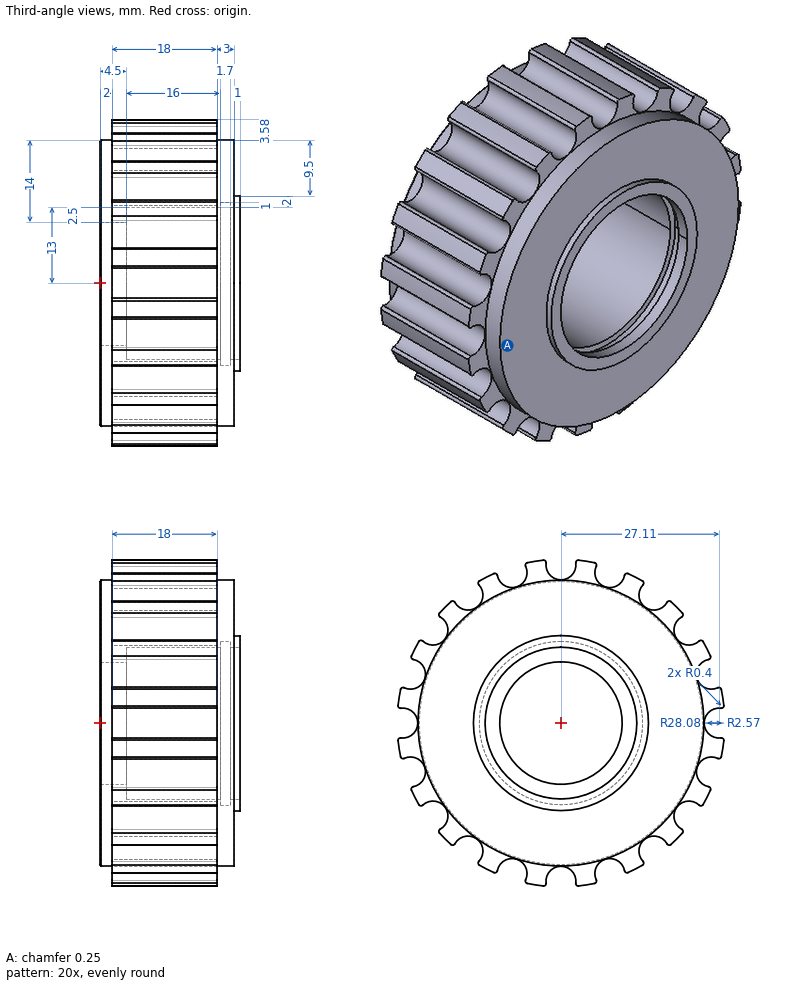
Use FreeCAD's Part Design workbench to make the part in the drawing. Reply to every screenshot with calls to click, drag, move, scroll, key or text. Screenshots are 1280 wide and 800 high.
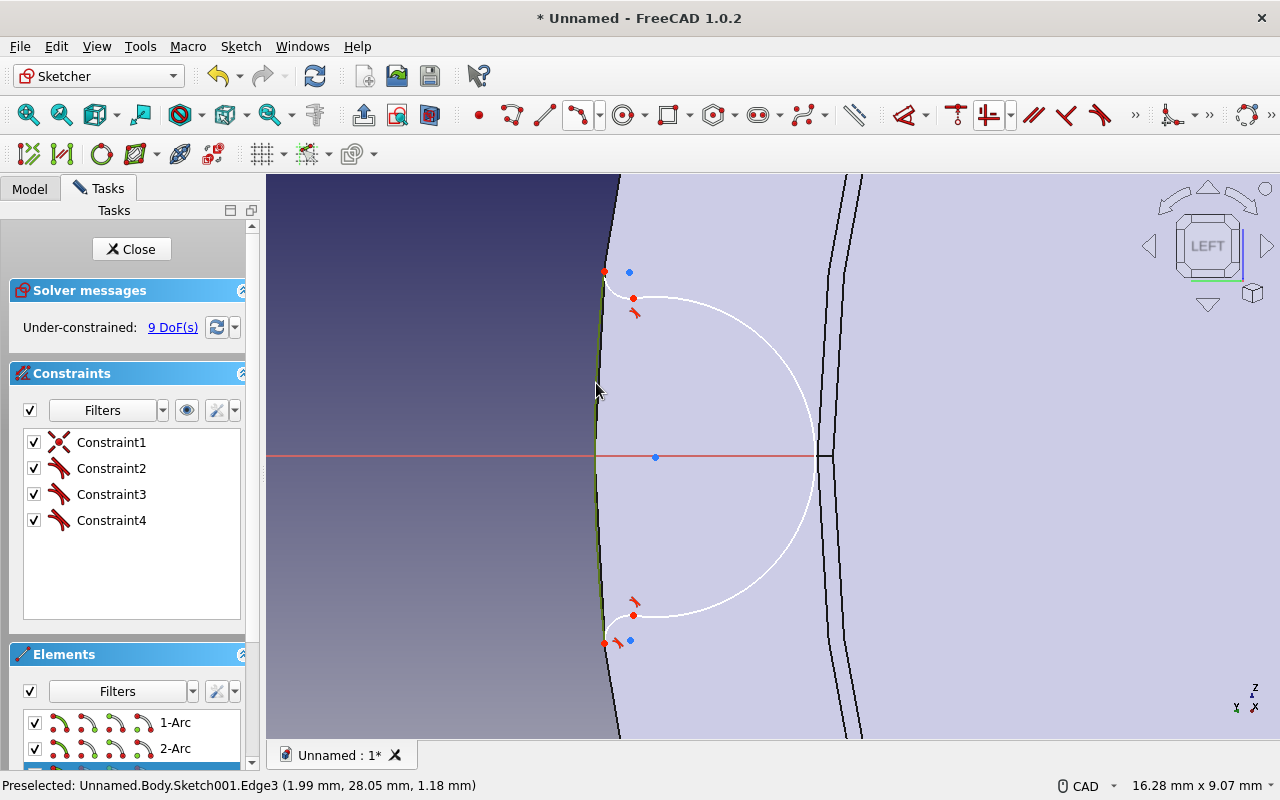
click(620, 297)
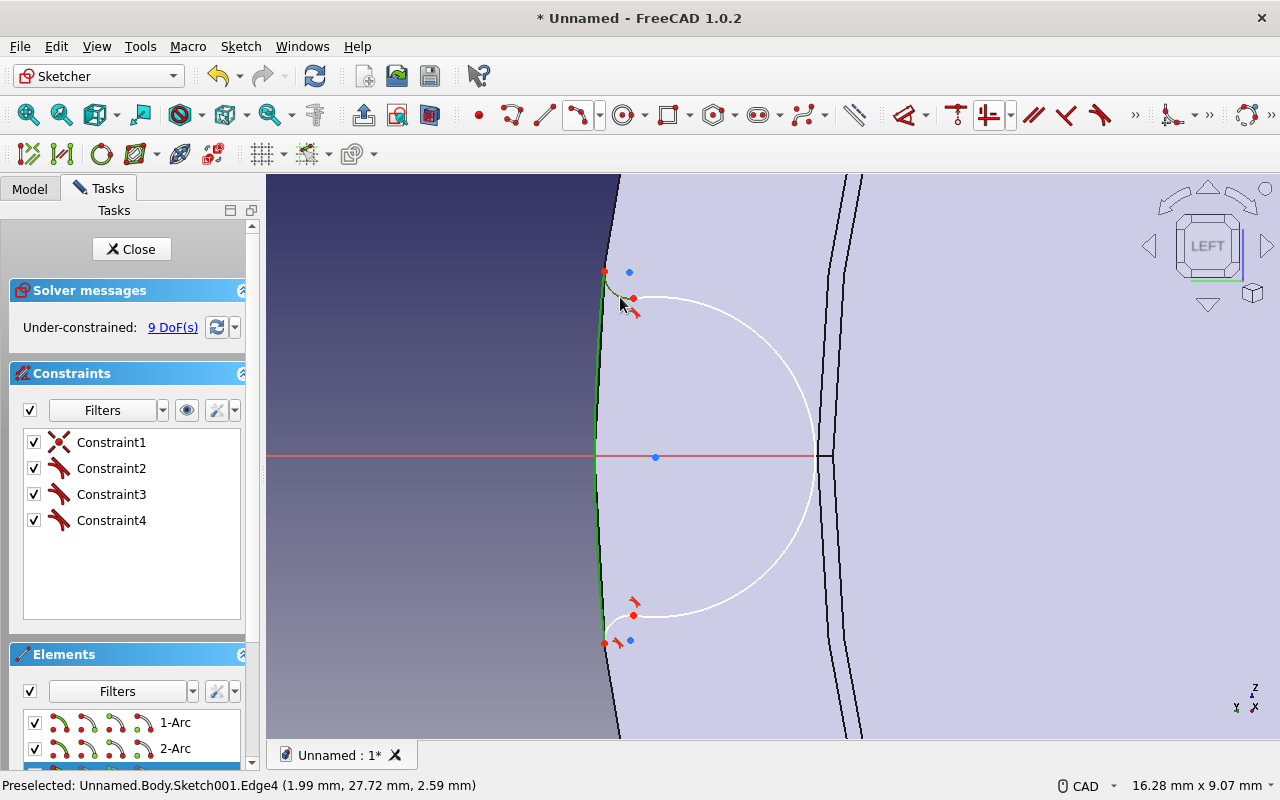
click(1100, 116)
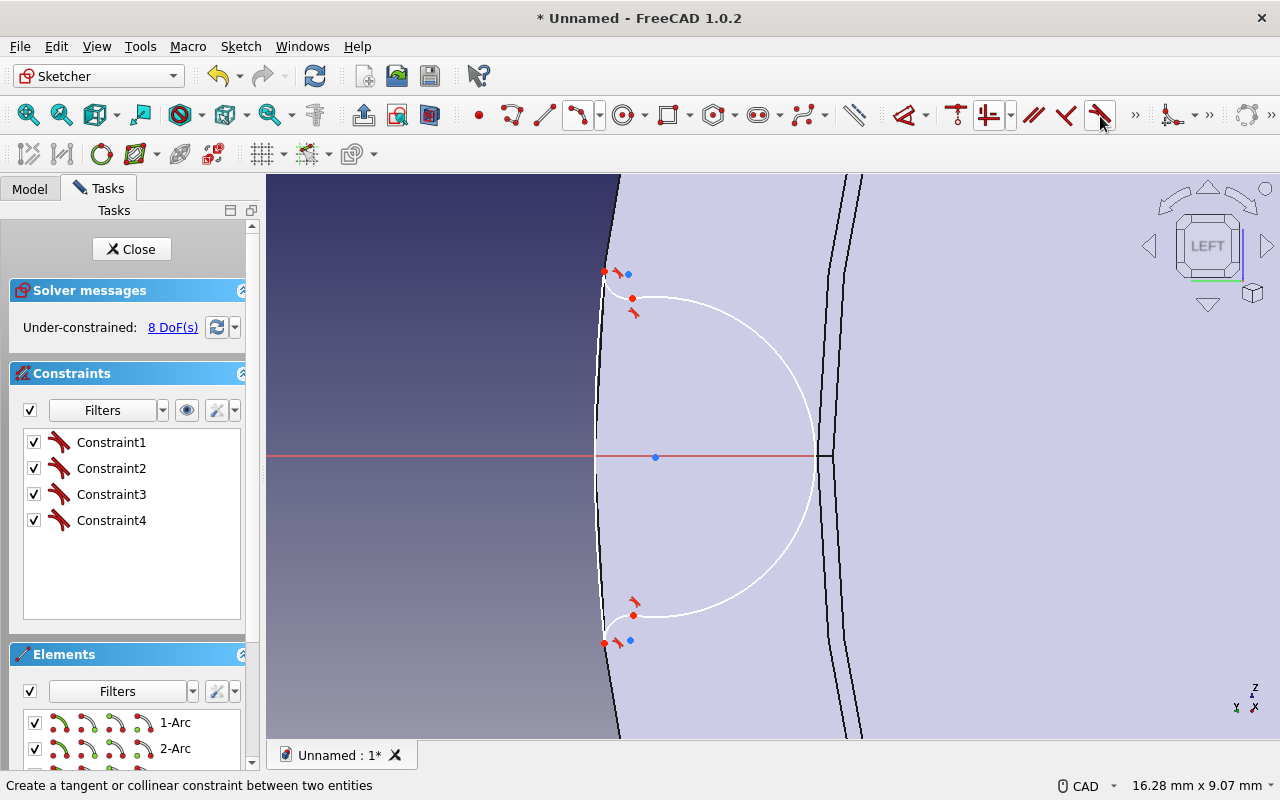
scroll(368, 457, down, 6)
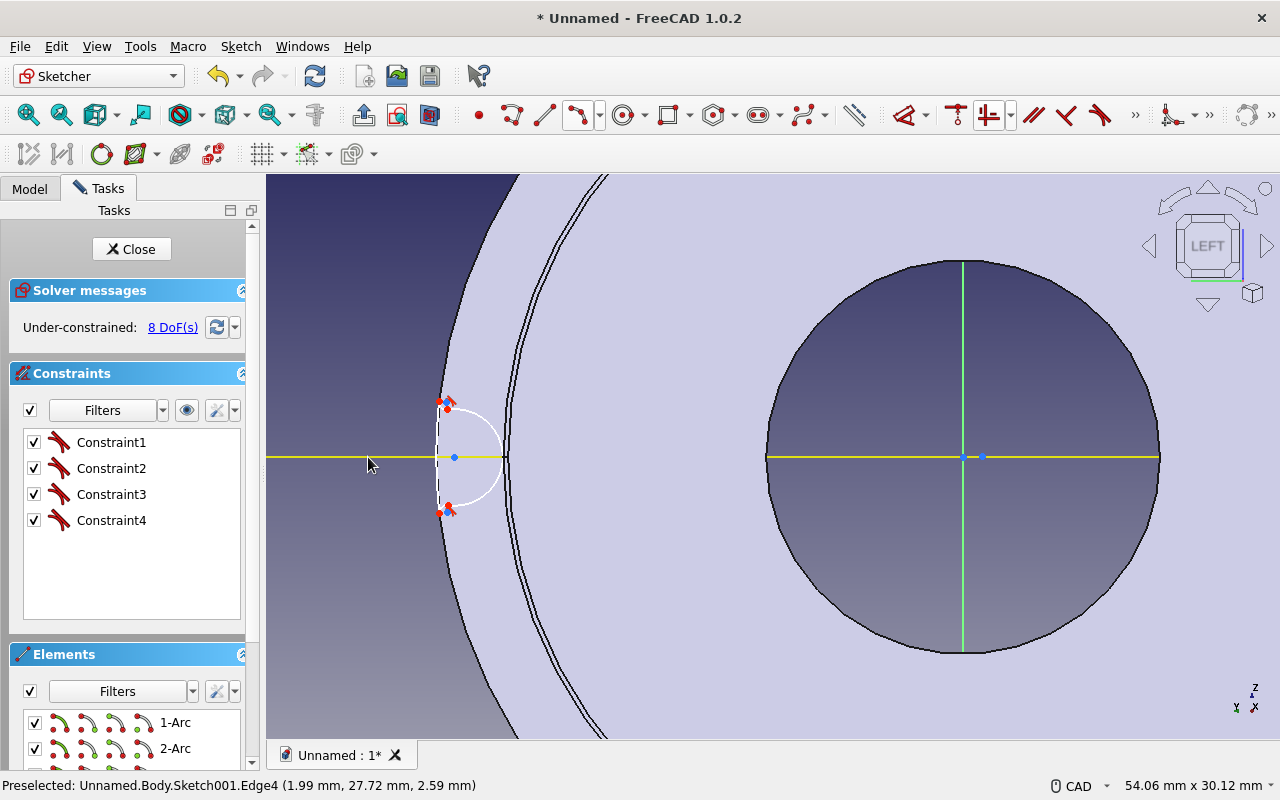
scroll(973, 457, up, 9)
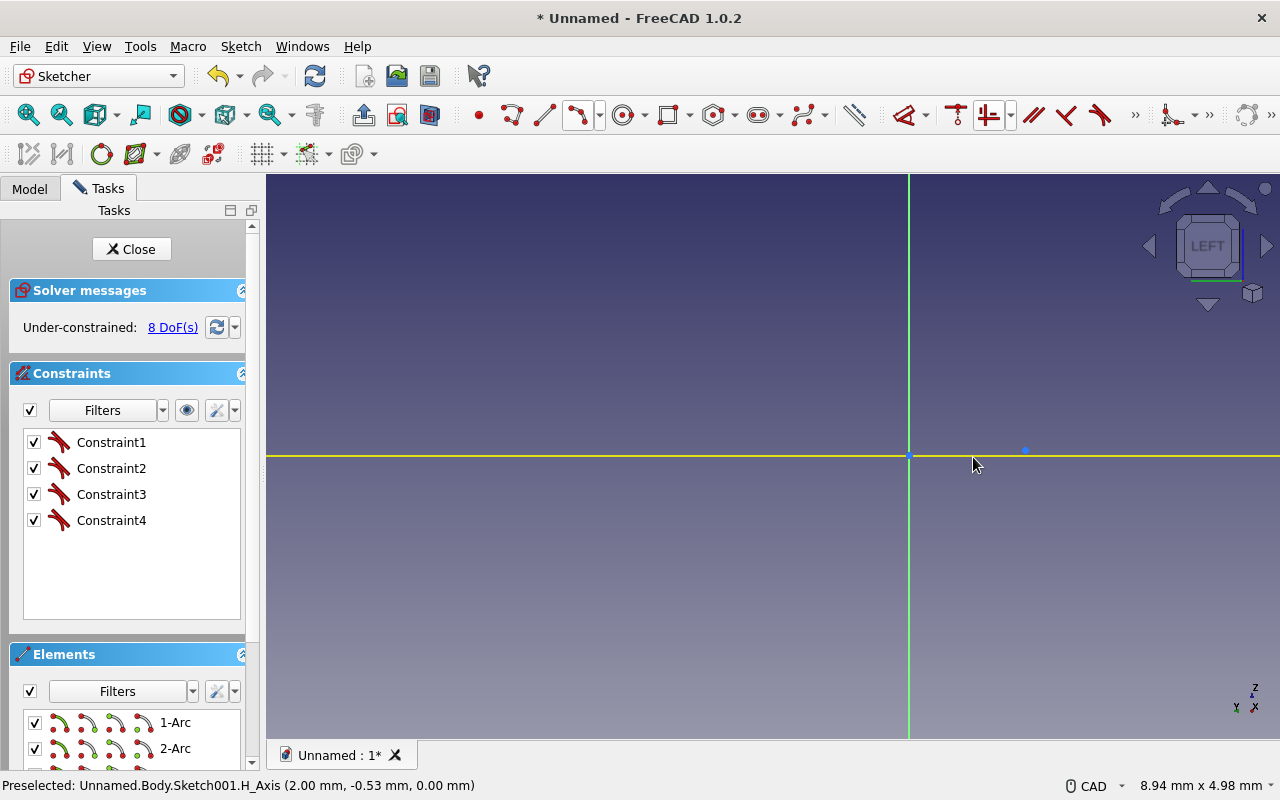
drag(899, 440, 1036, 466)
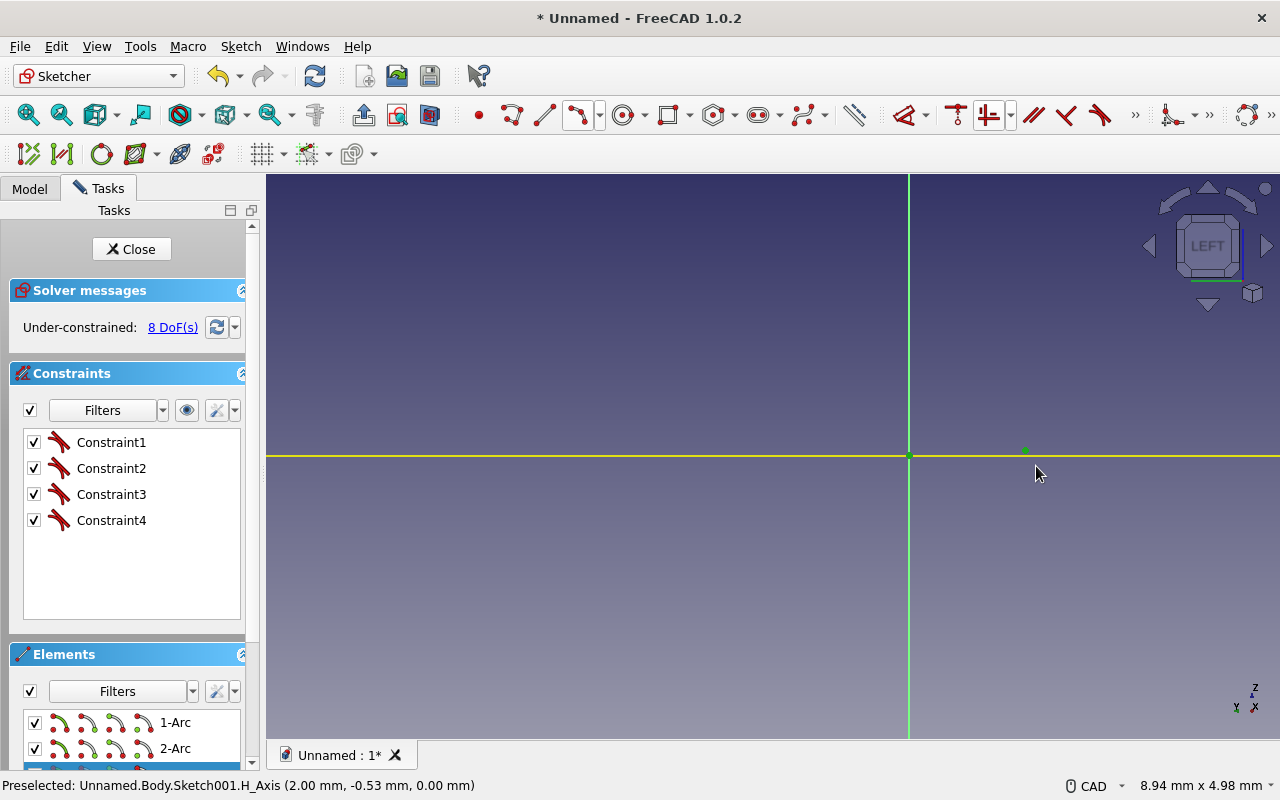
click(956, 116)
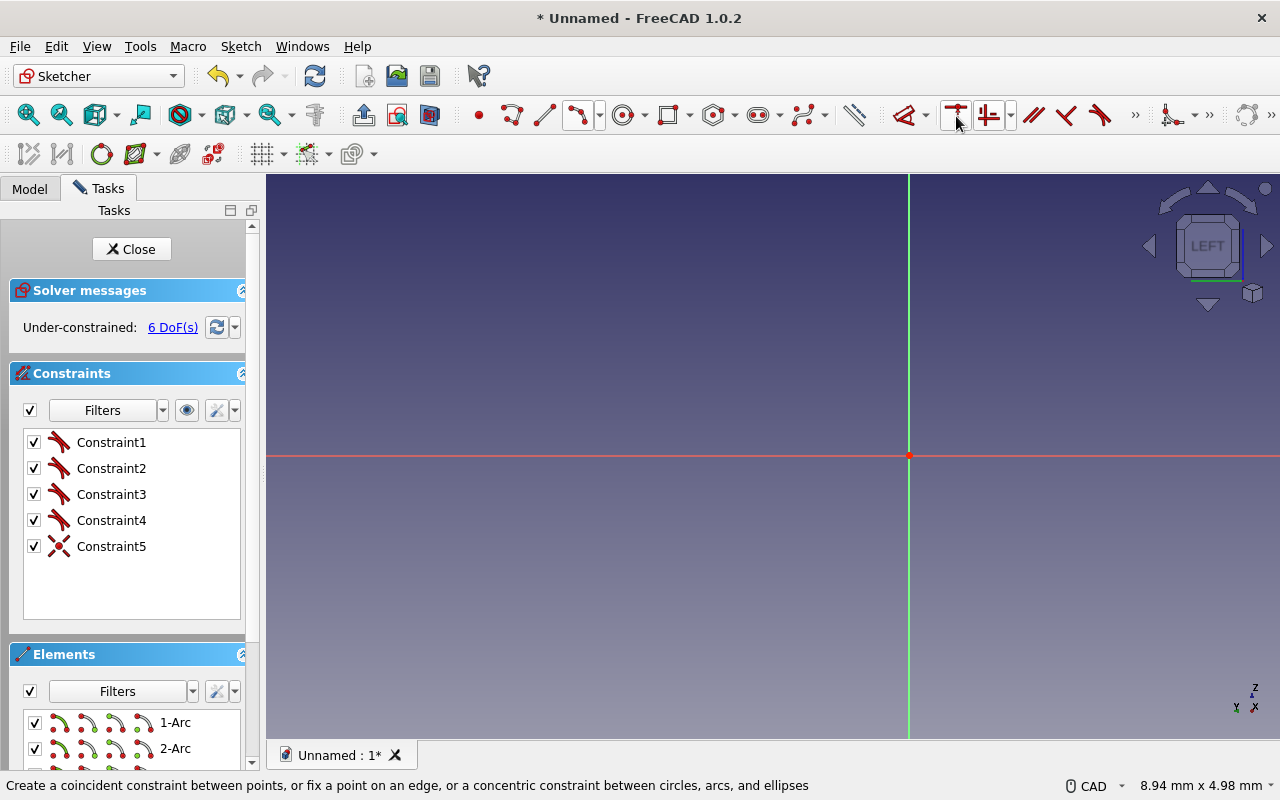
scroll(704, 456, down, 5)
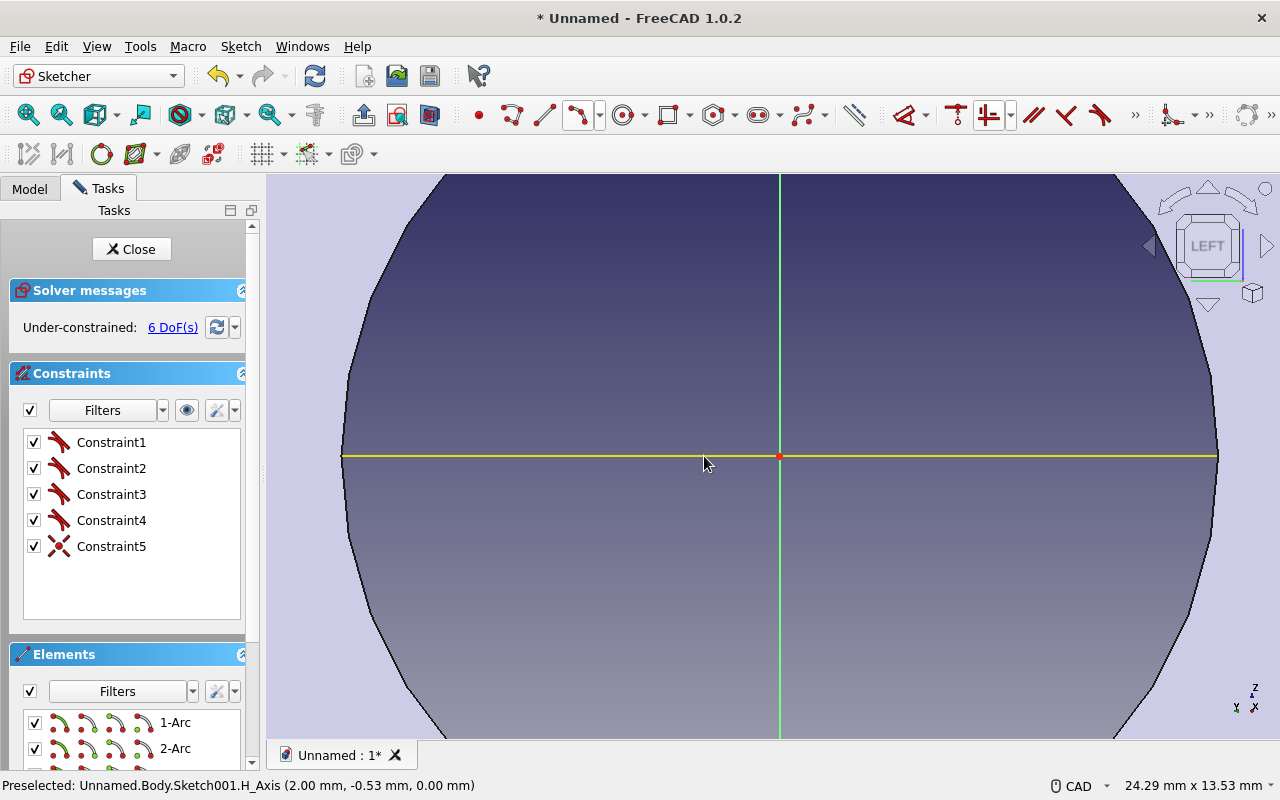
scroll(704, 456, down, 5)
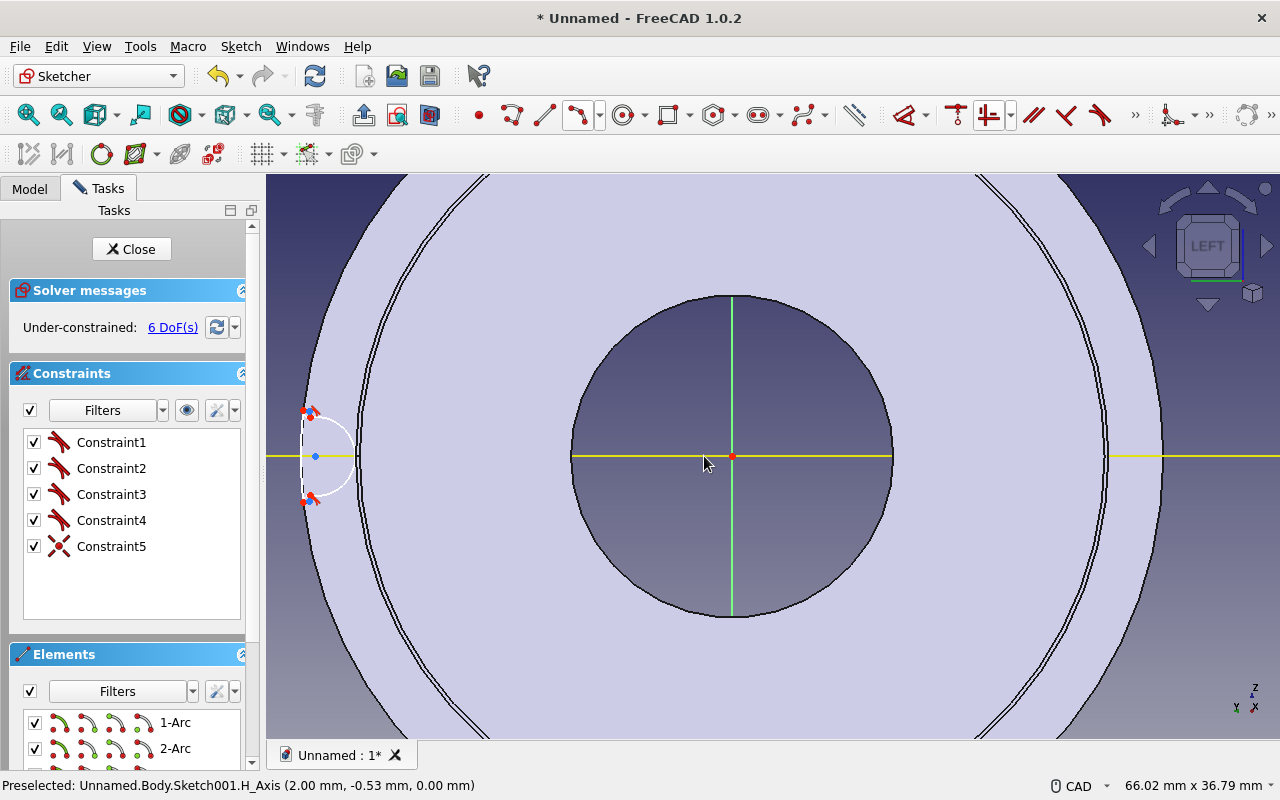
scroll(294, 456, up, 7)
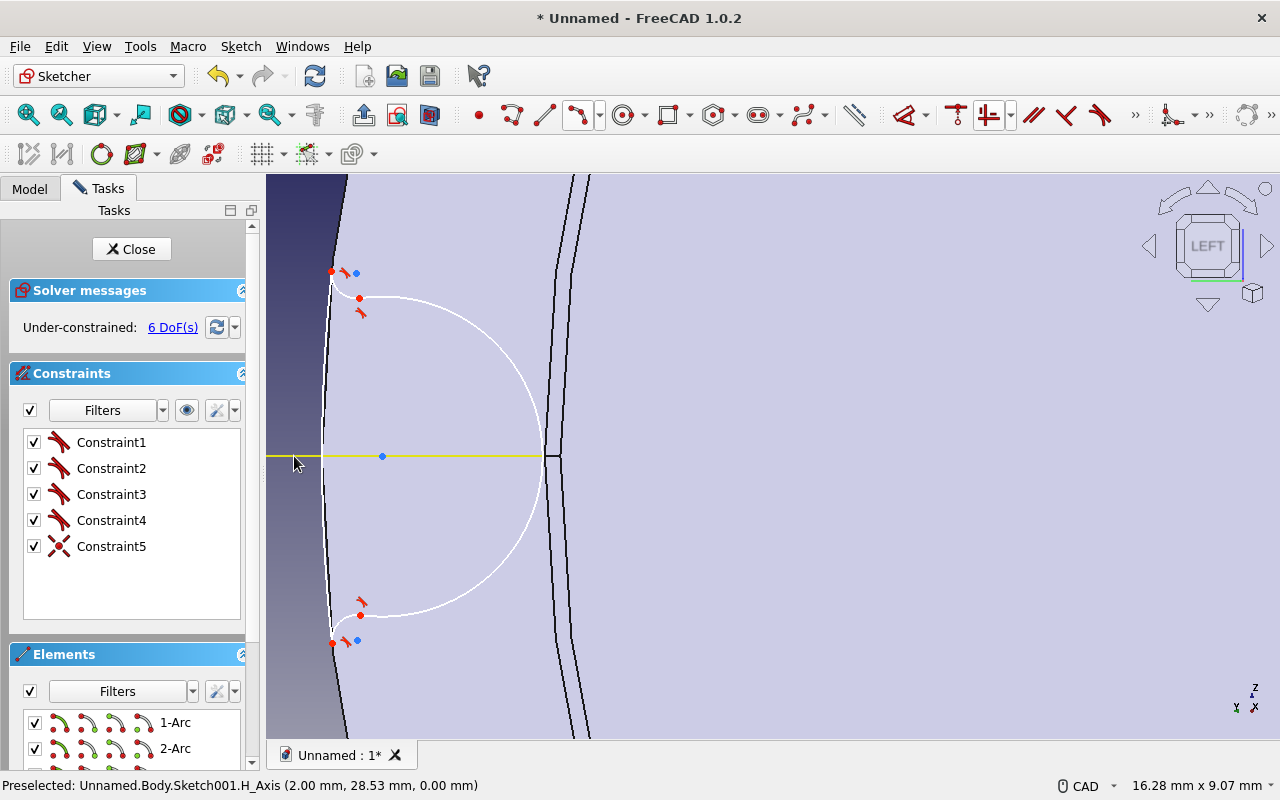
click(347, 617)